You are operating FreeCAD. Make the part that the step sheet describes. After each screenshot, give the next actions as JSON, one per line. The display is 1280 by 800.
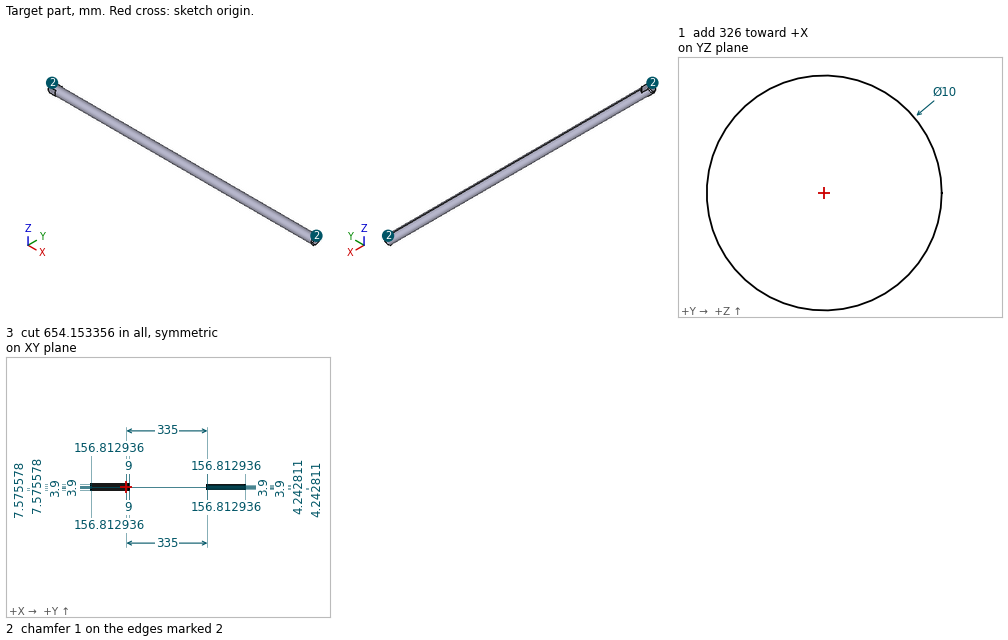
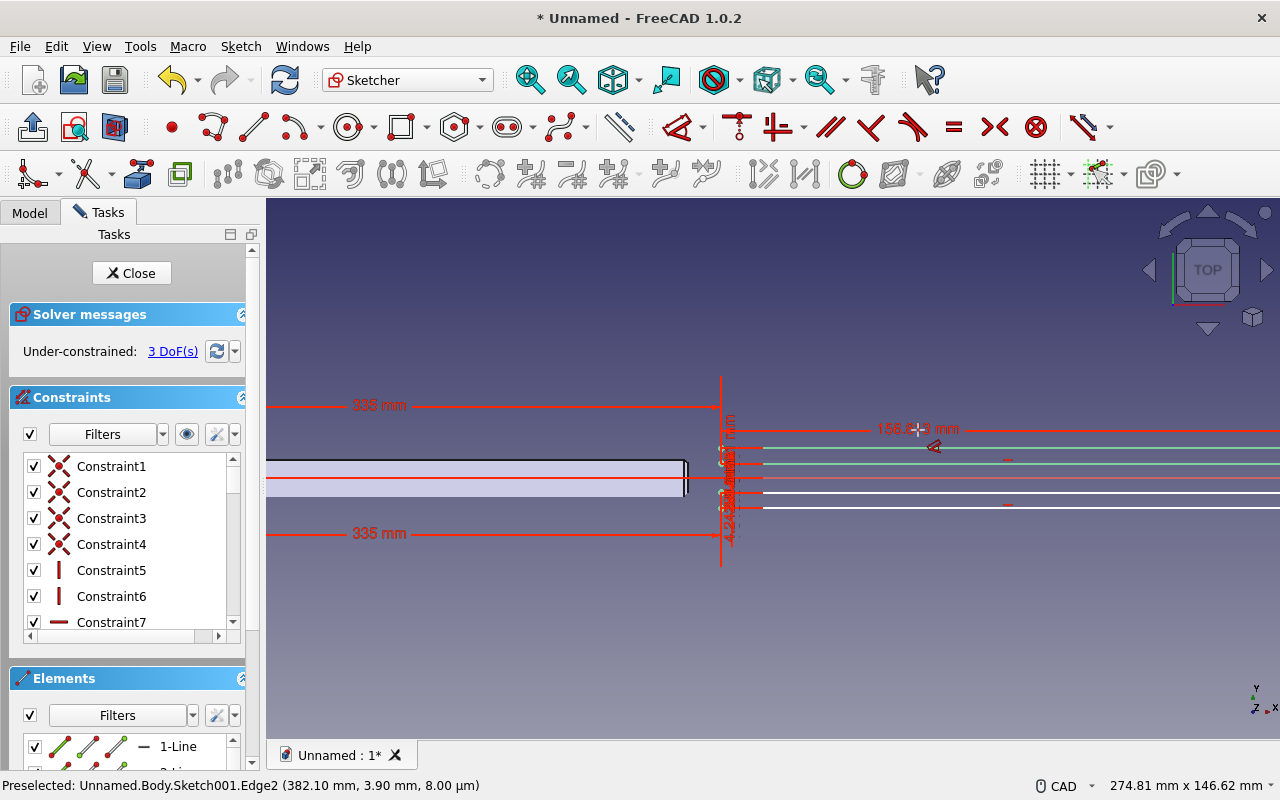
{"action": "left_click", "coordinate": [895, 508]}
{"action": "left_click", "coordinate": [918, 542]}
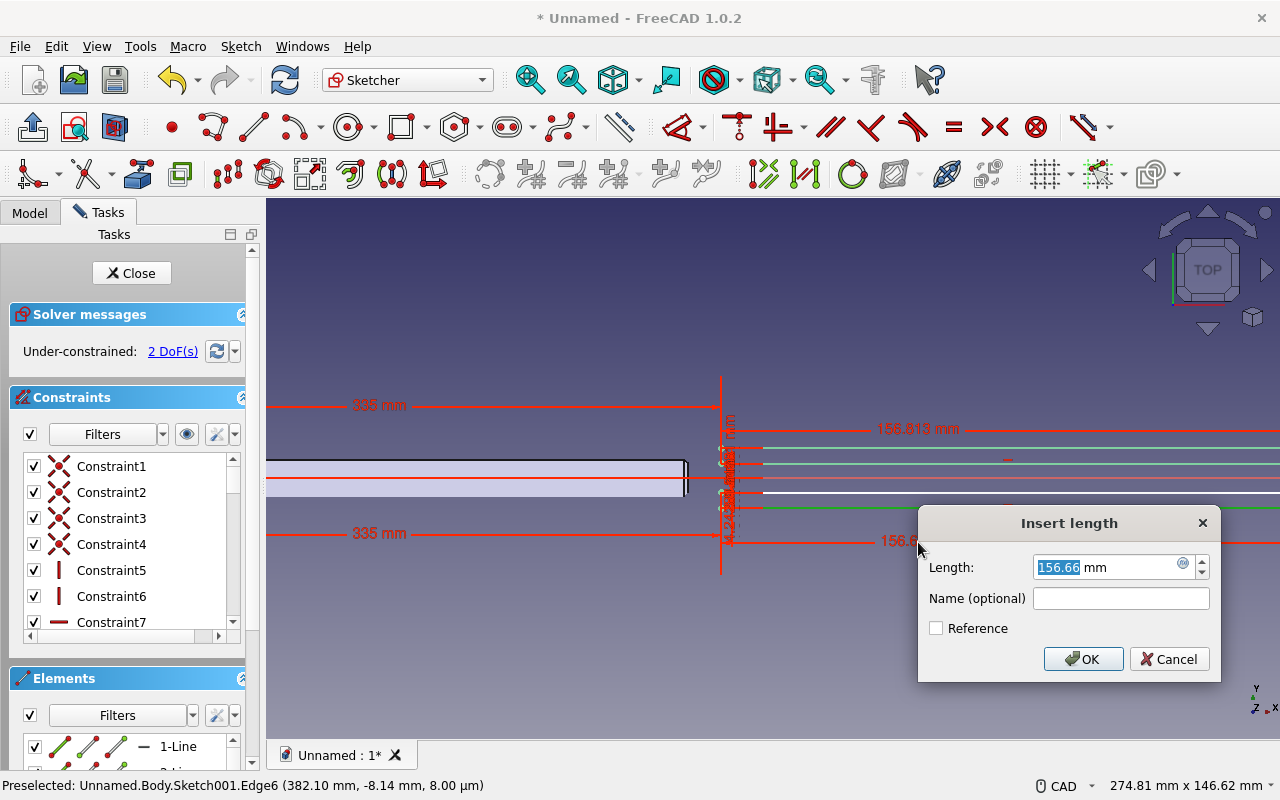
{"action": "type", "text": "156.812936"}
{"action": "key", "text": "Return"}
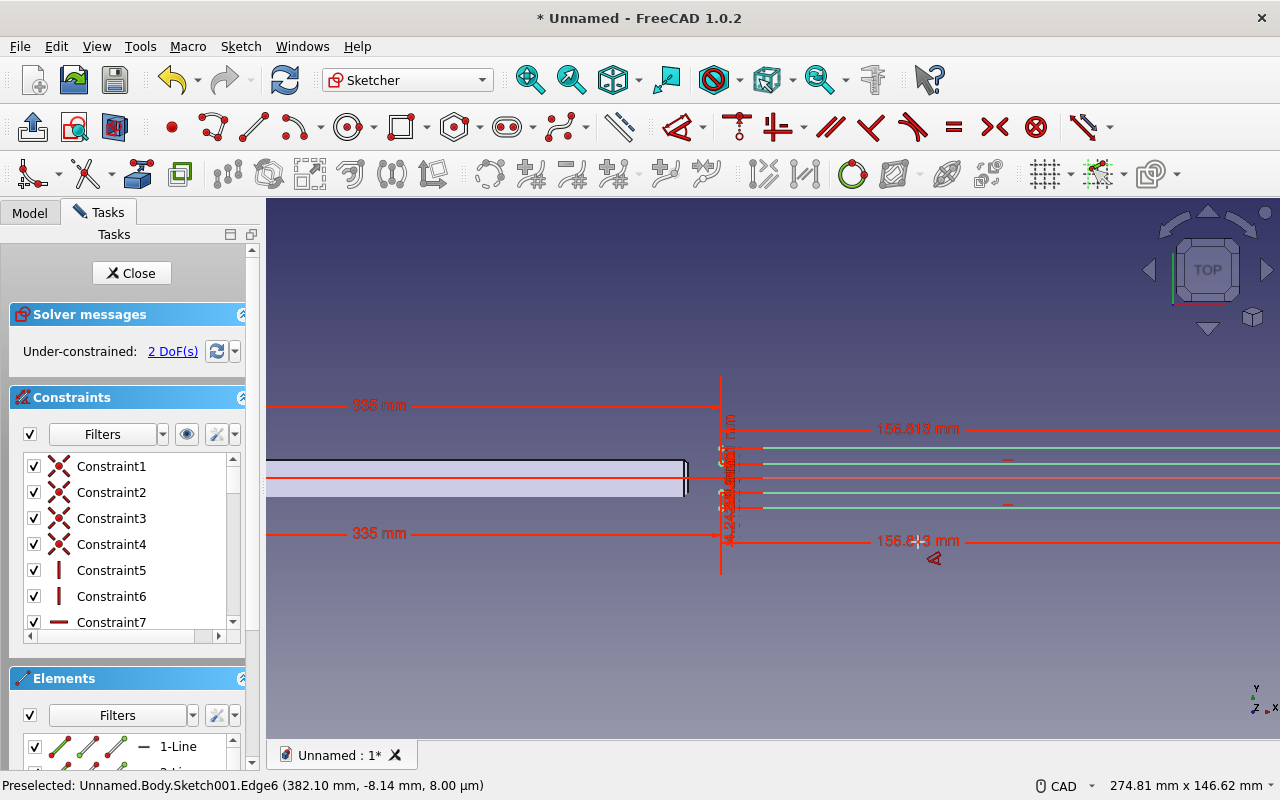
{"action": "scroll", "coordinate": [896, 465], "scroll_direction": "down", "scroll_amount": 7}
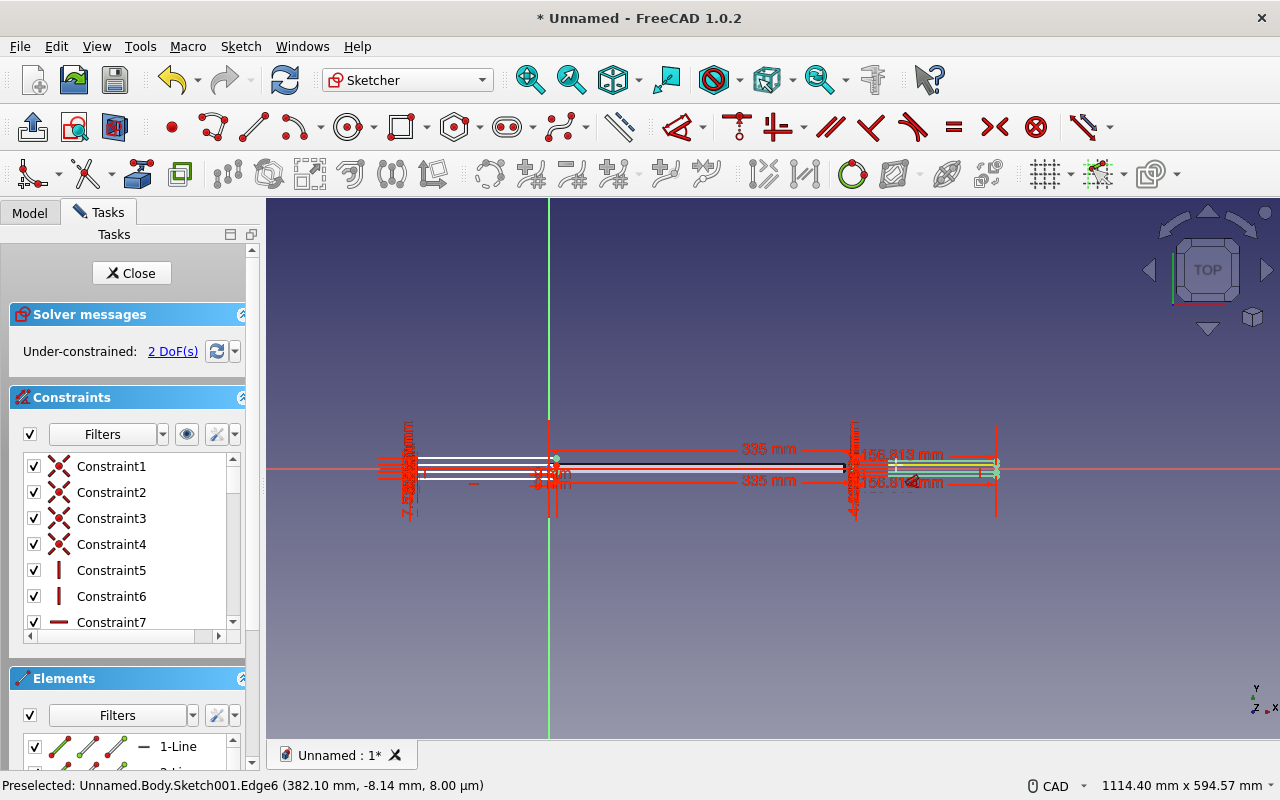
{"action": "scroll", "coordinate": [457, 465], "scroll_direction": "up", "scroll_amount": 7}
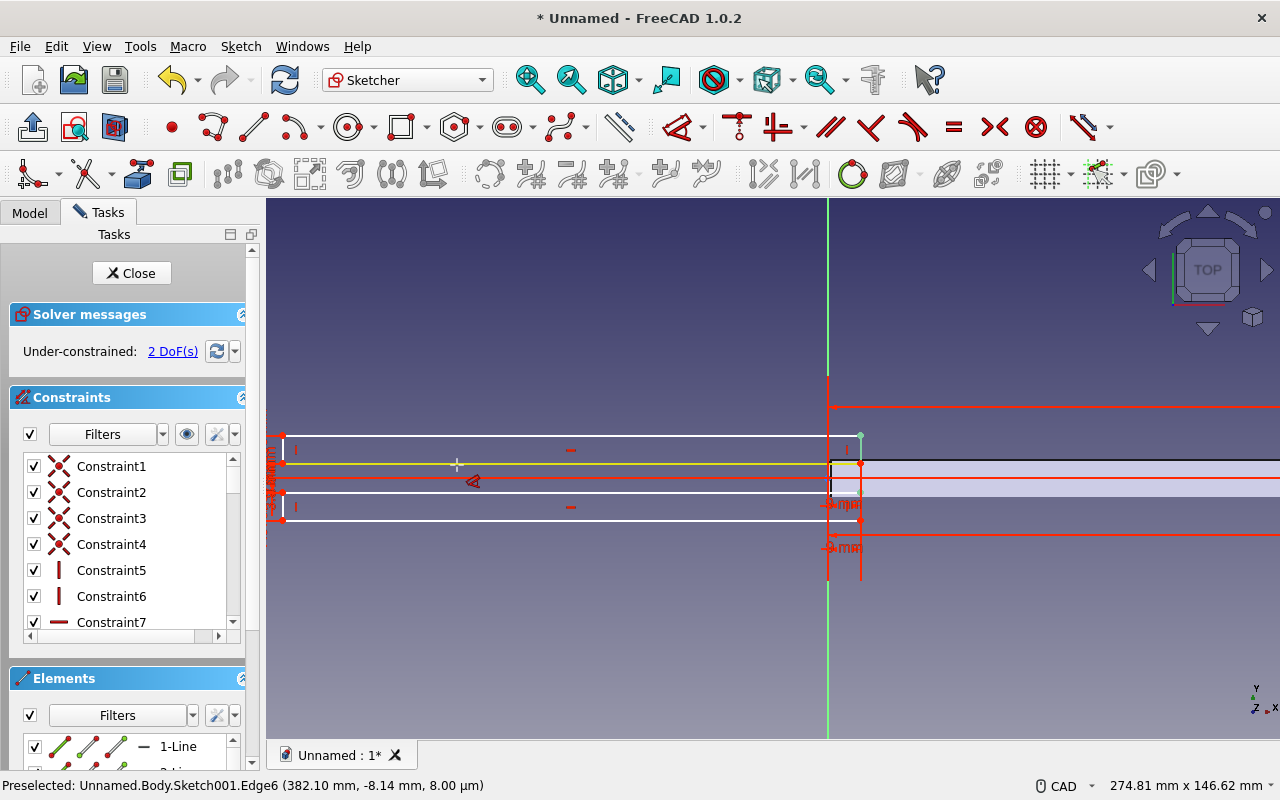
{"action": "left_click", "coordinate": [456, 464]}
{"action": "left_click", "coordinate": [577, 406]}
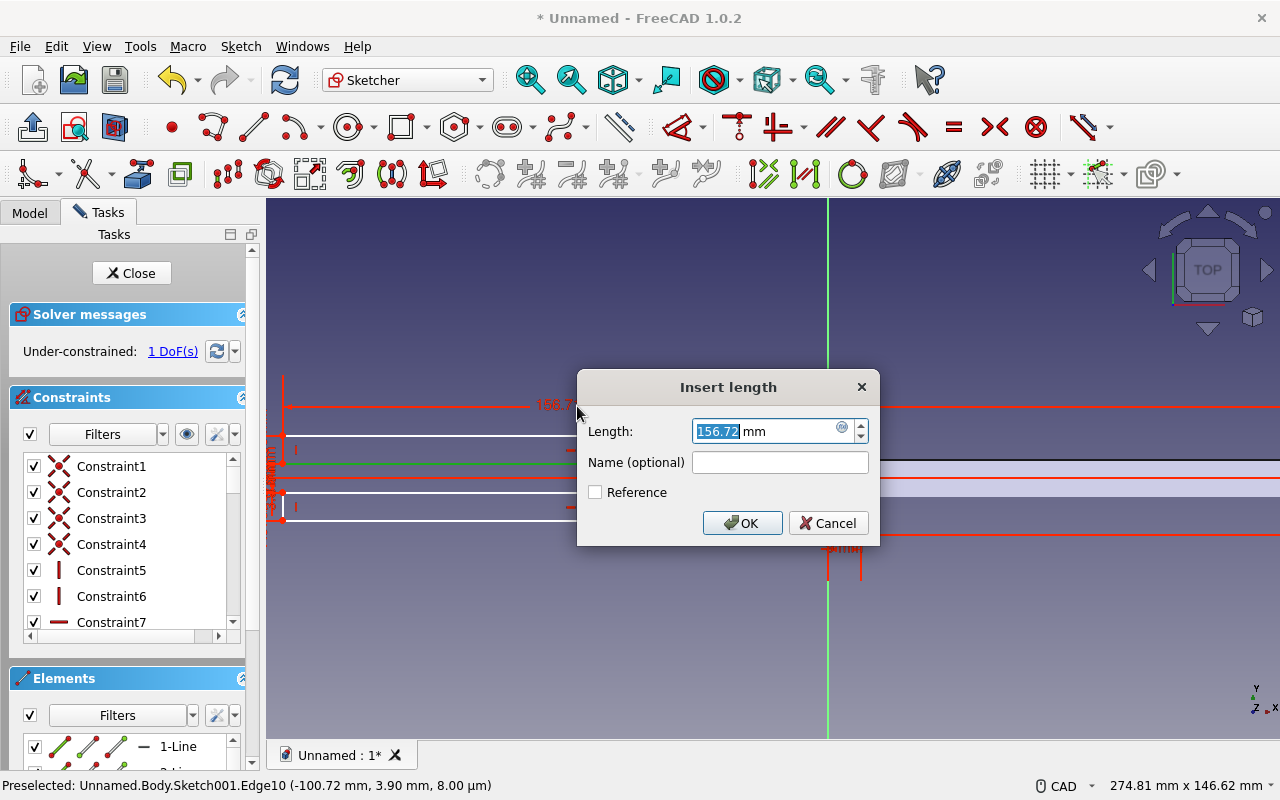
{"action": "type", "text": "156.812936"}
{"action": "key", "text": "Return"}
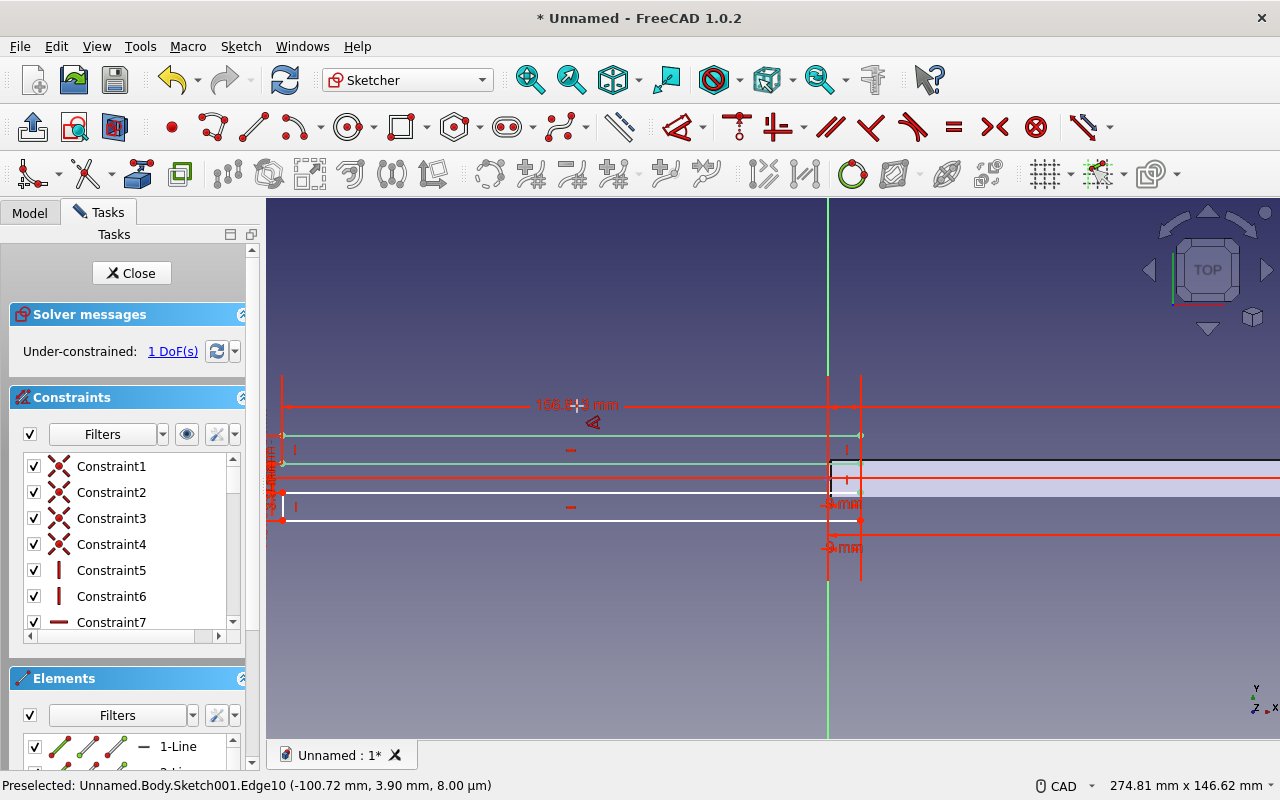
{"action": "left_click", "coordinate": [456, 521]}
{"action": "left_click", "coordinate": [577, 555]}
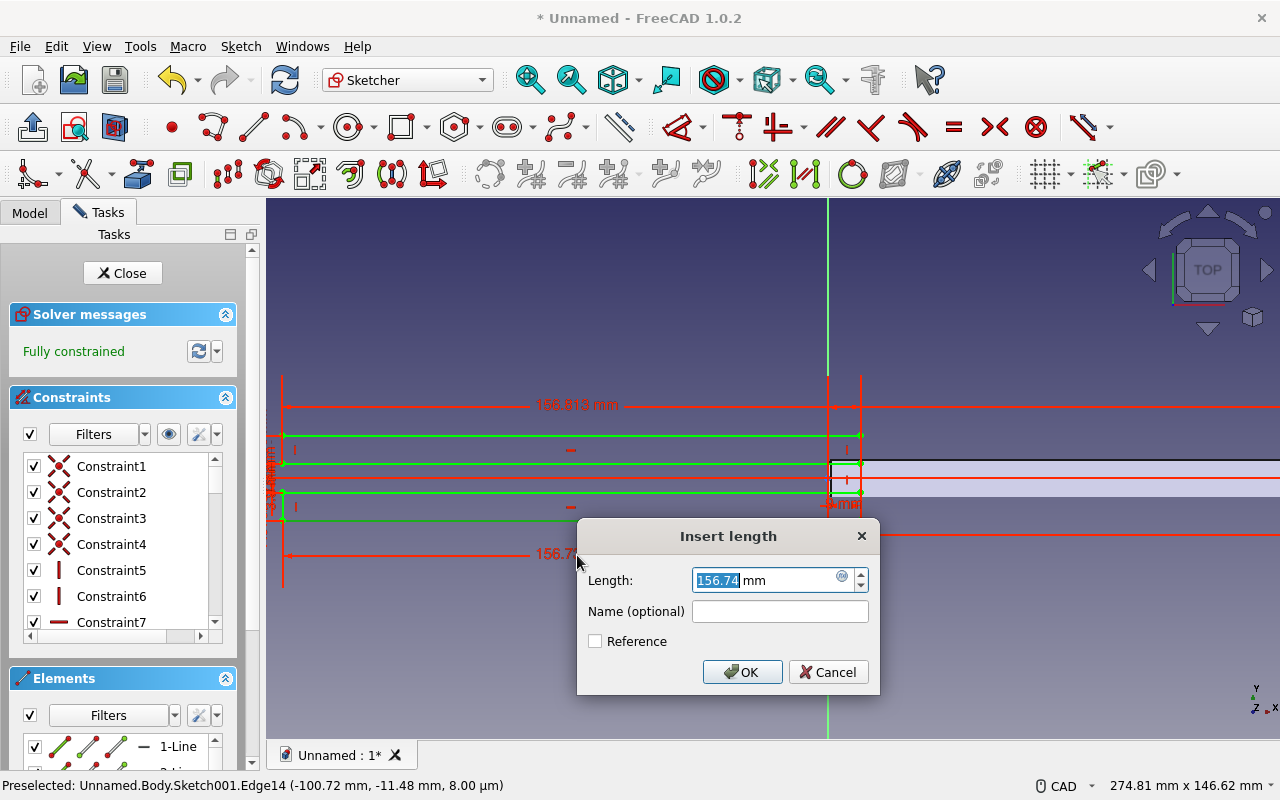
{"action": "type", "text": "156.812936"}
{"action": "key", "text": "Return"}
{"action": "key", "text": "Escape"}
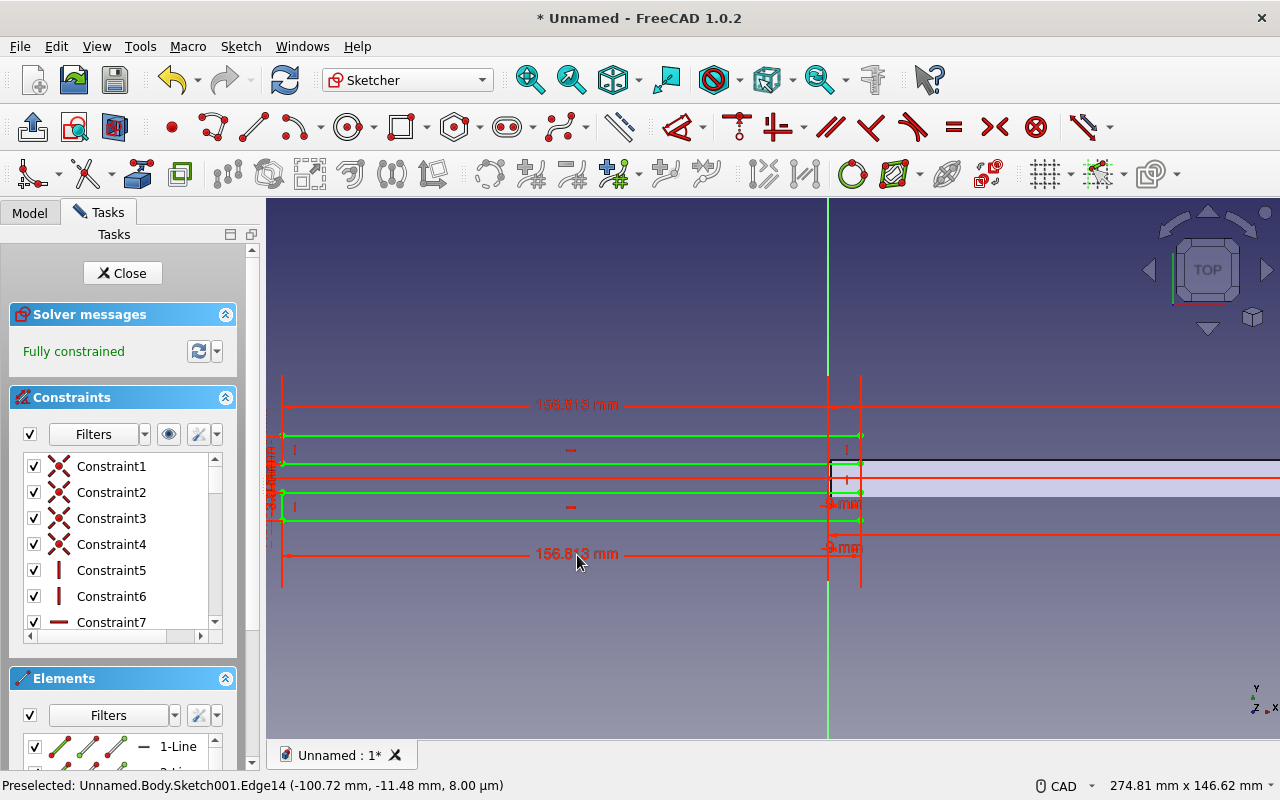
{"action": "left_click", "coordinate": [123, 273]}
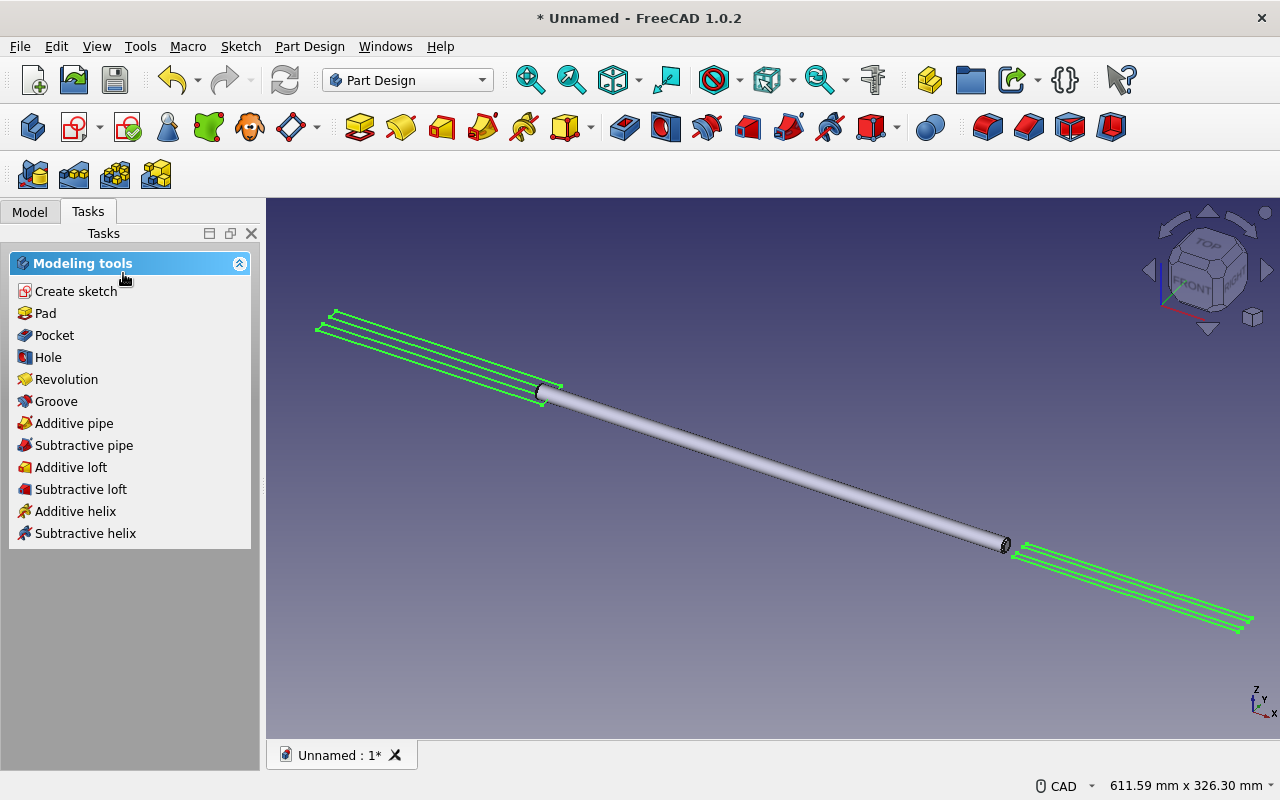
{"action": "left_click", "coordinate": [625, 128]}